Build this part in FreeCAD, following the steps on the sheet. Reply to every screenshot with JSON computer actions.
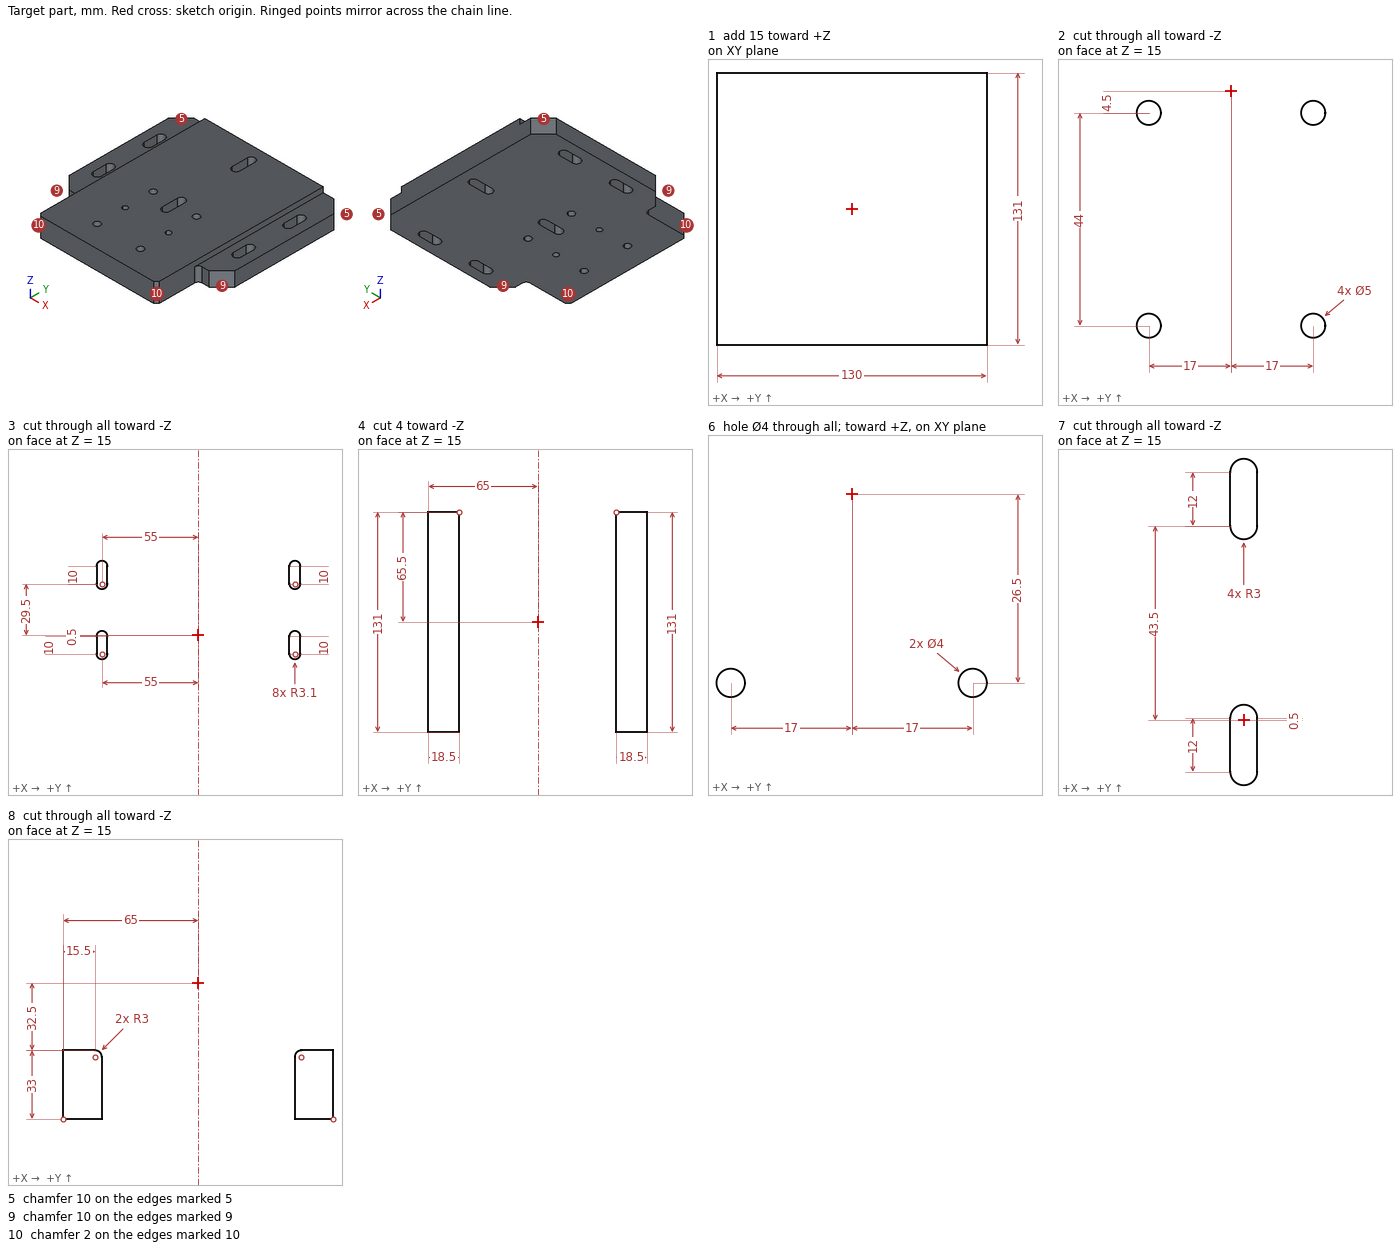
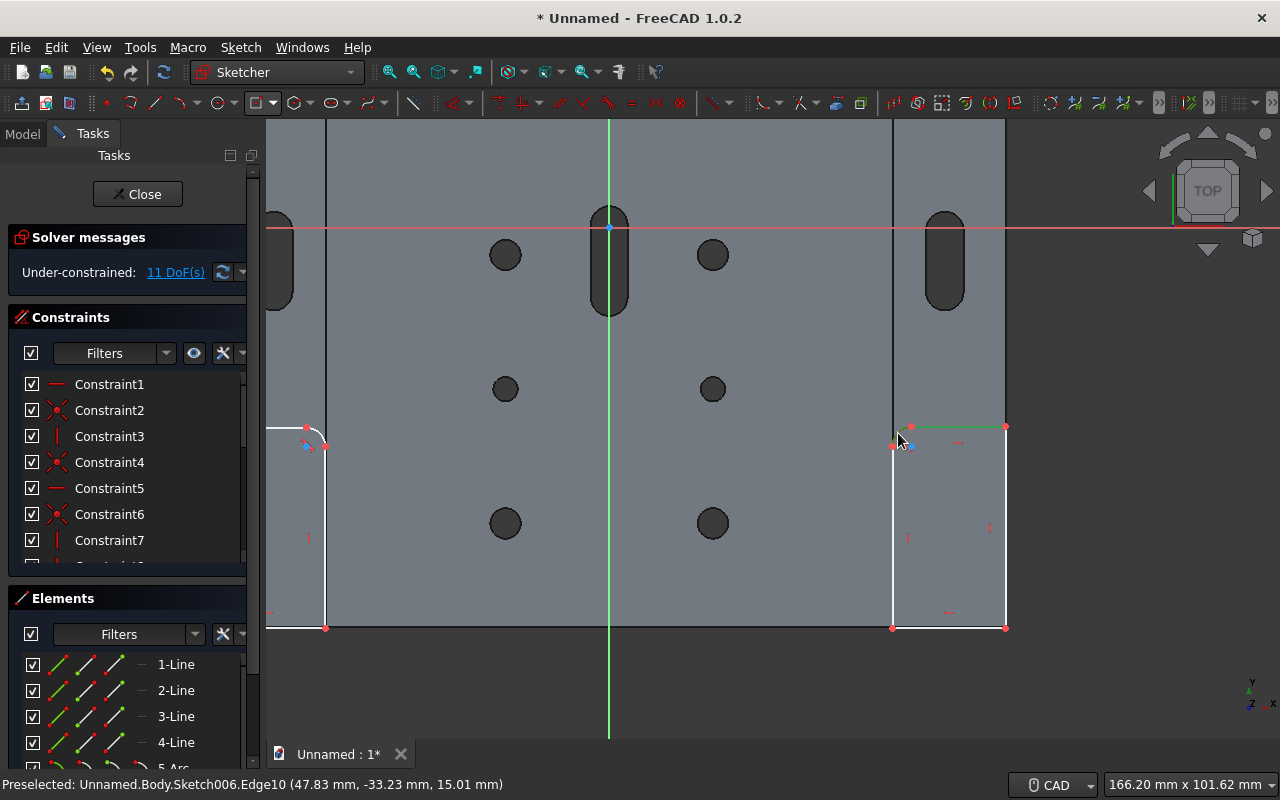
{"action": "key", "text": "t"}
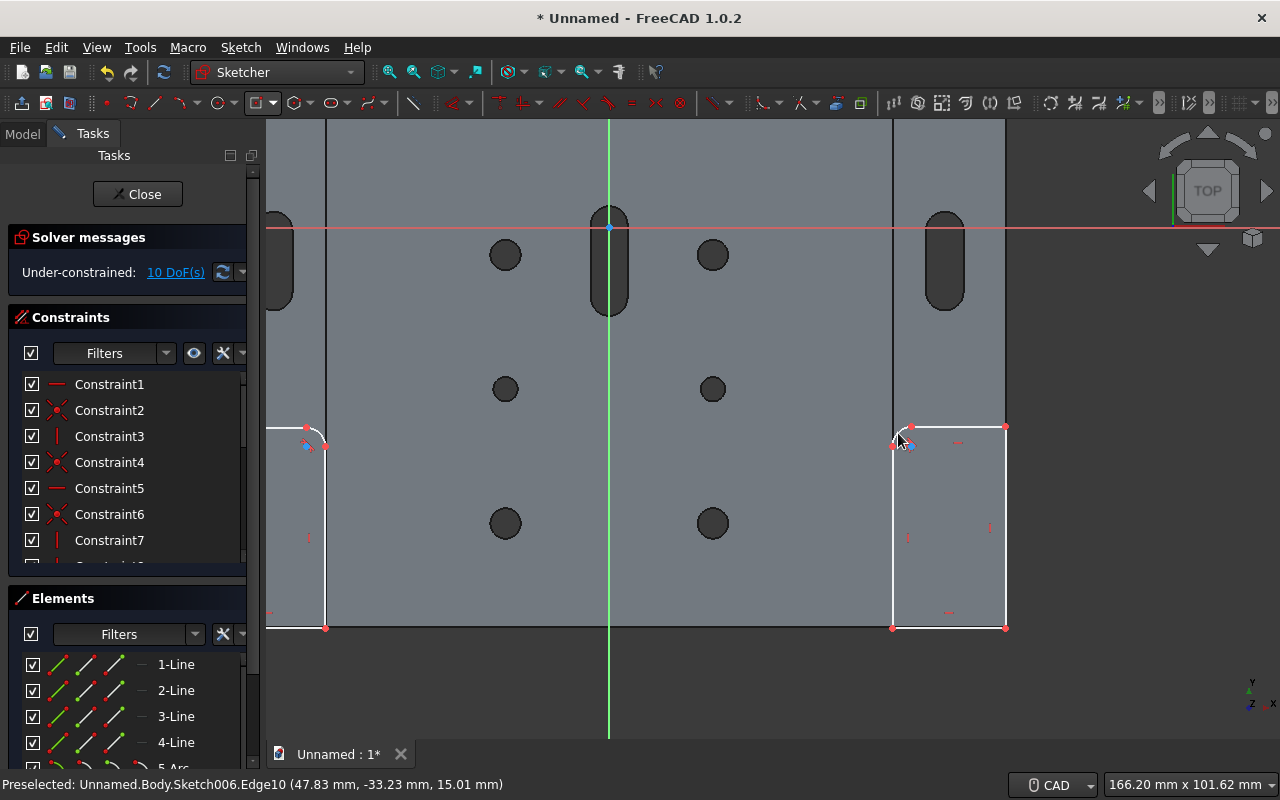
{"action": "left_click", "coordinate": [320, 433]}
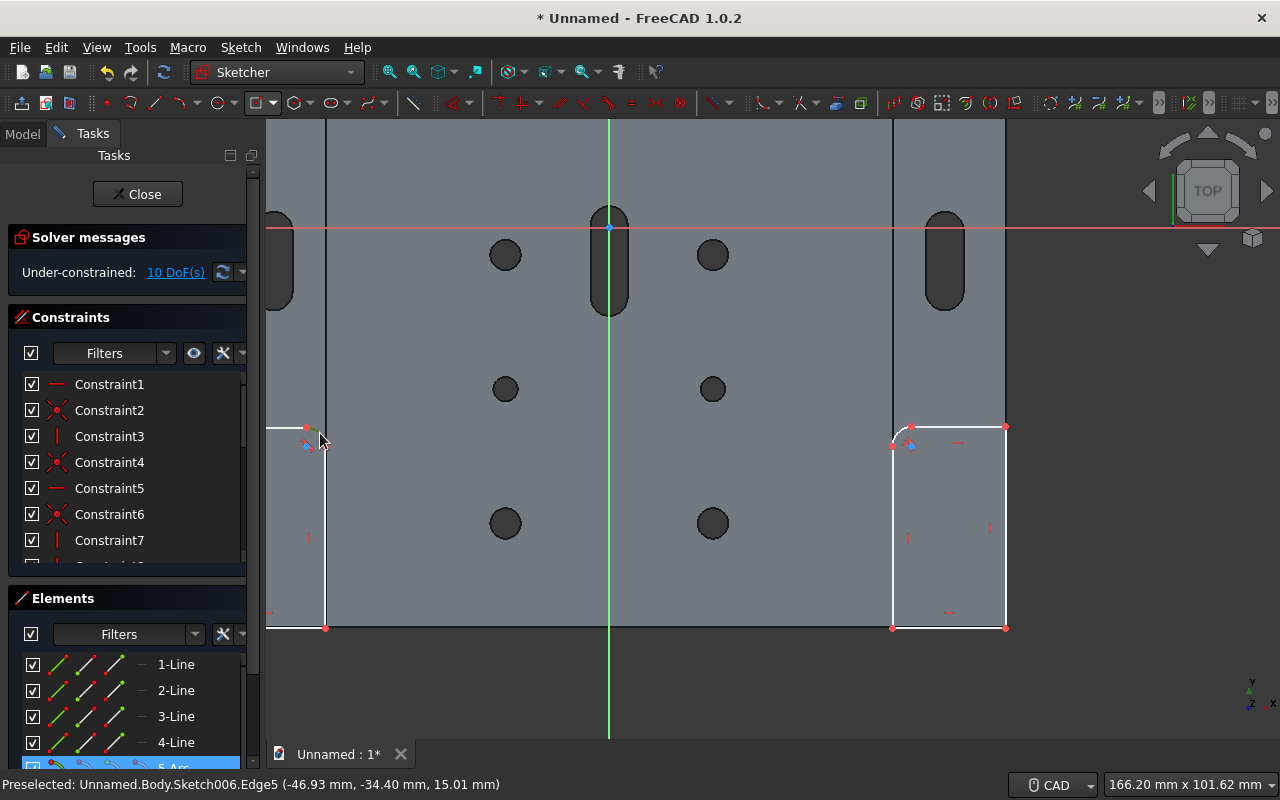
{"action": "scroll", "coordinate": [903, 429], "scroll_direction": "up", "scroll_amount": 3}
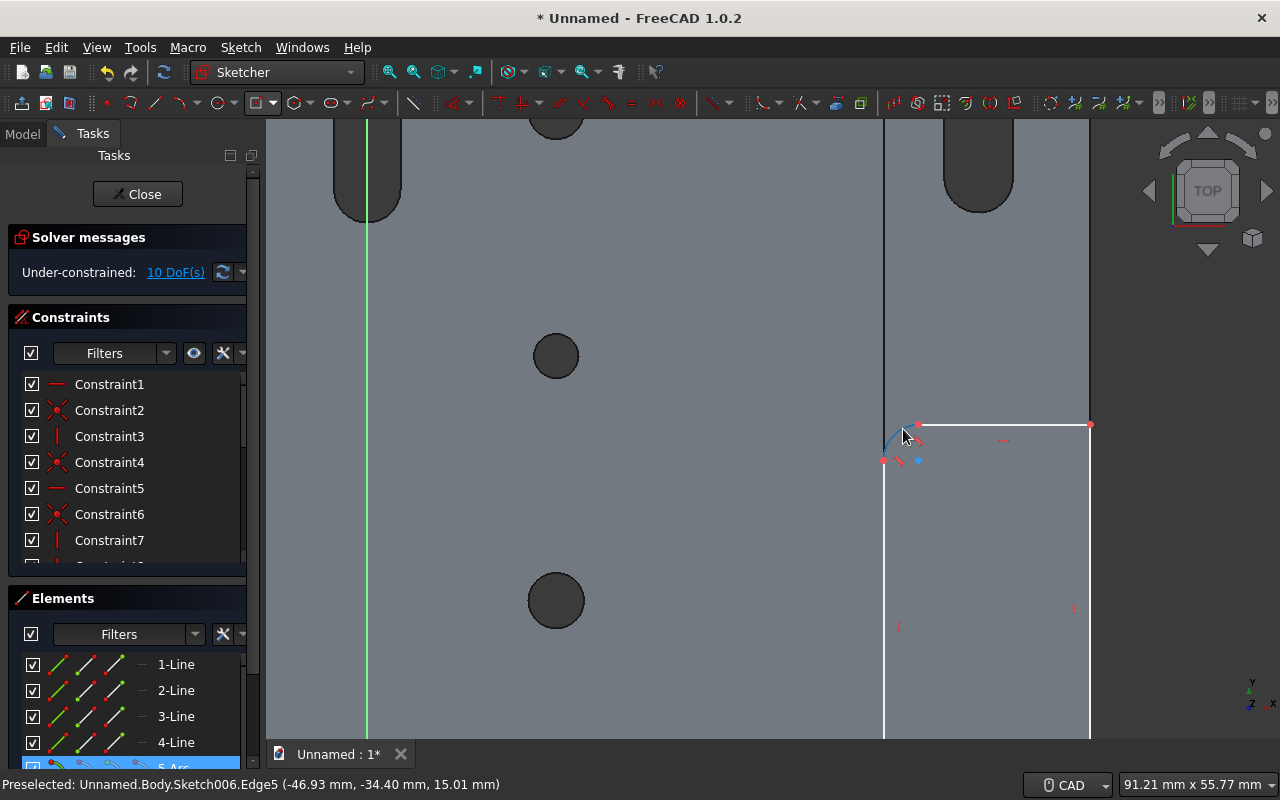
{"action": "left_click", "coordinate": [903, 429]}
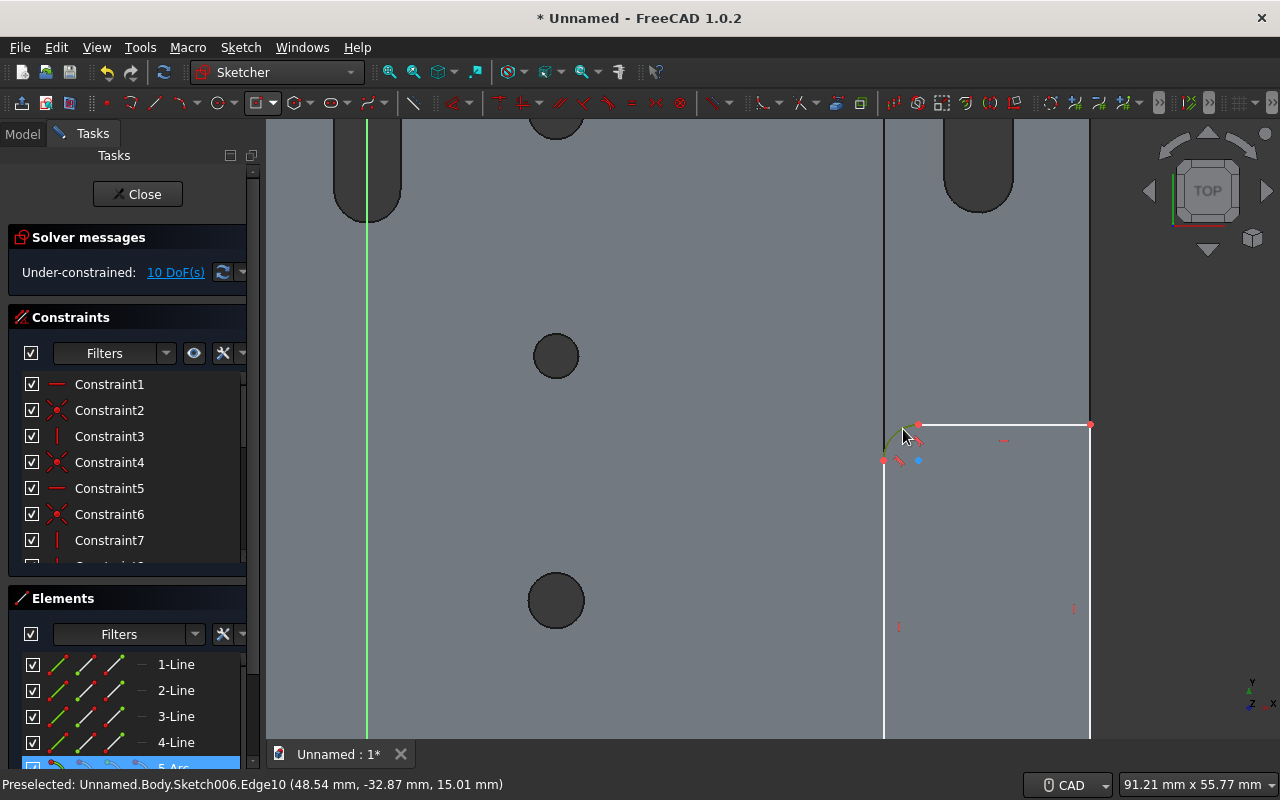
{"action": "key", "text": "e"}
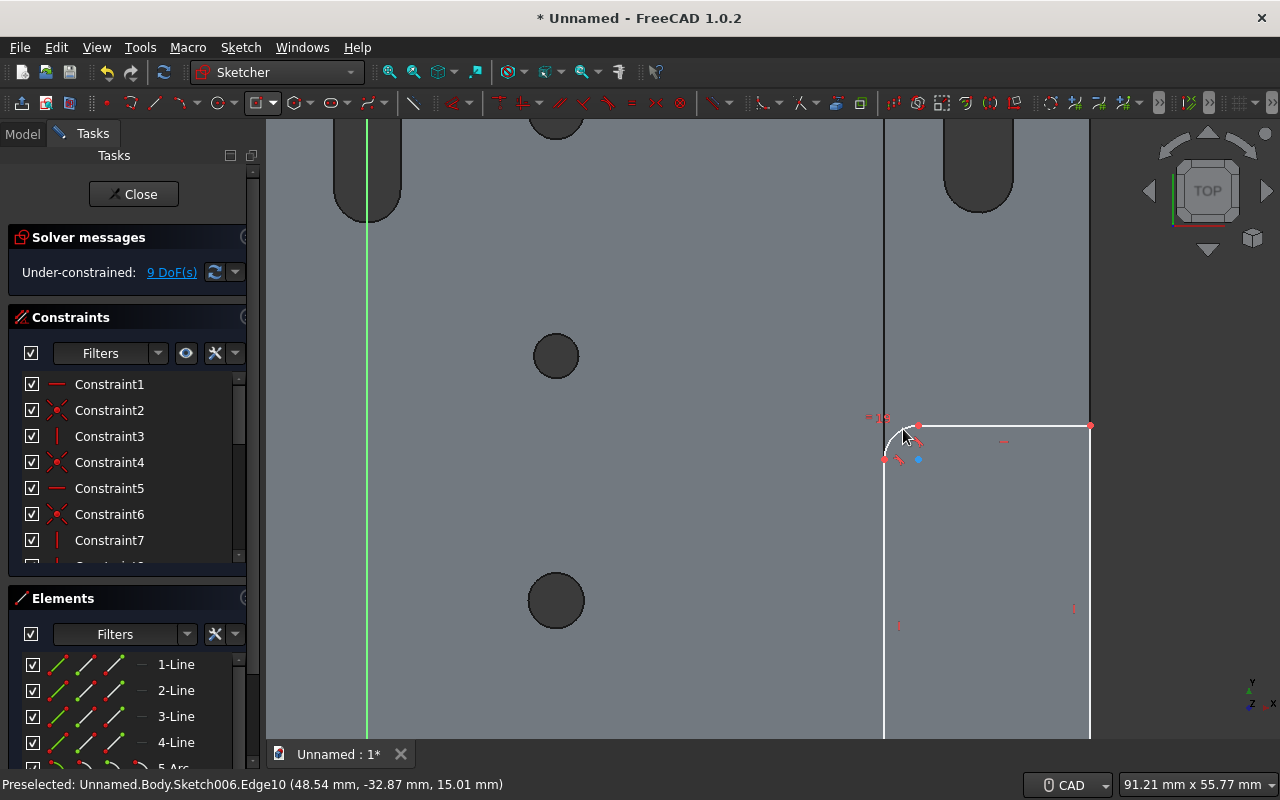
{"action": "scroll", "coordinate": [901, 431], "scroll_direction": "down", "scroll_amount": 5}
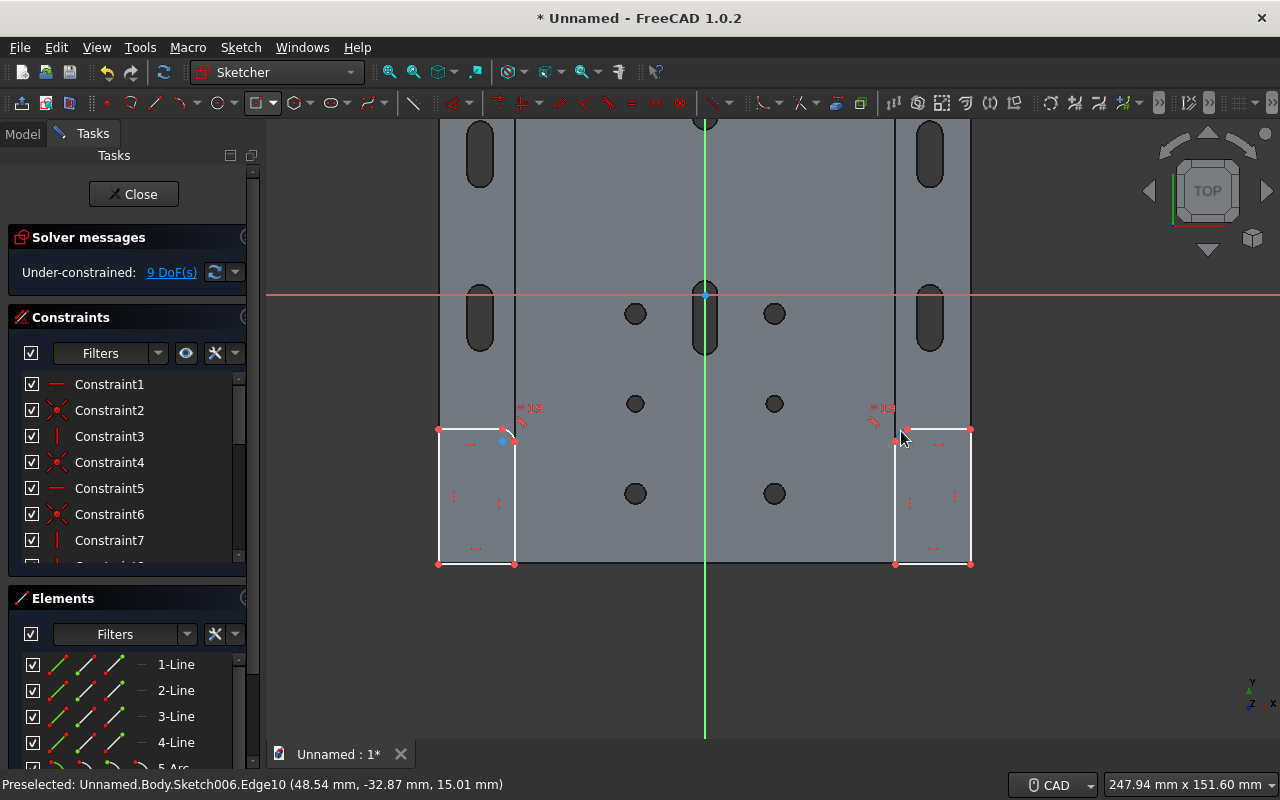
{"action": "left_click", "coordinate": [502, 442]}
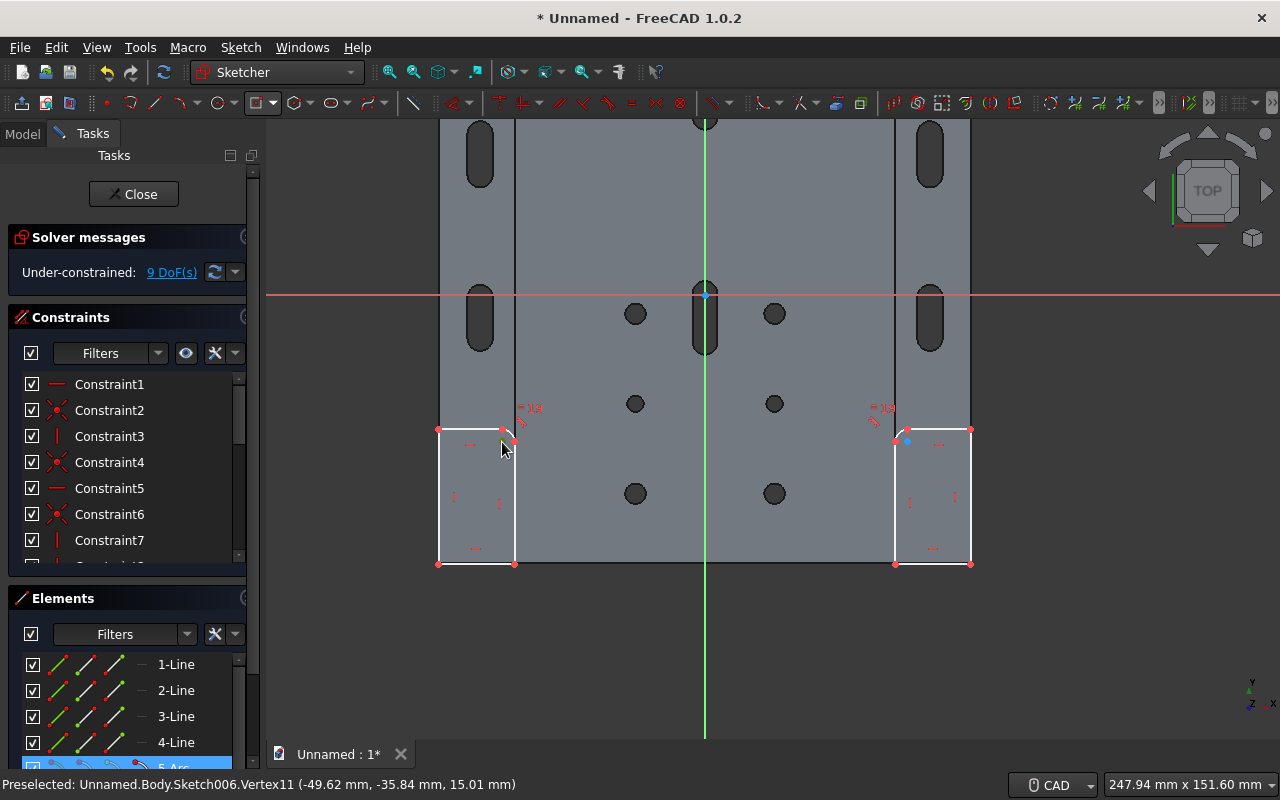
{"action": "left_click", "coordinate": [908, 442]}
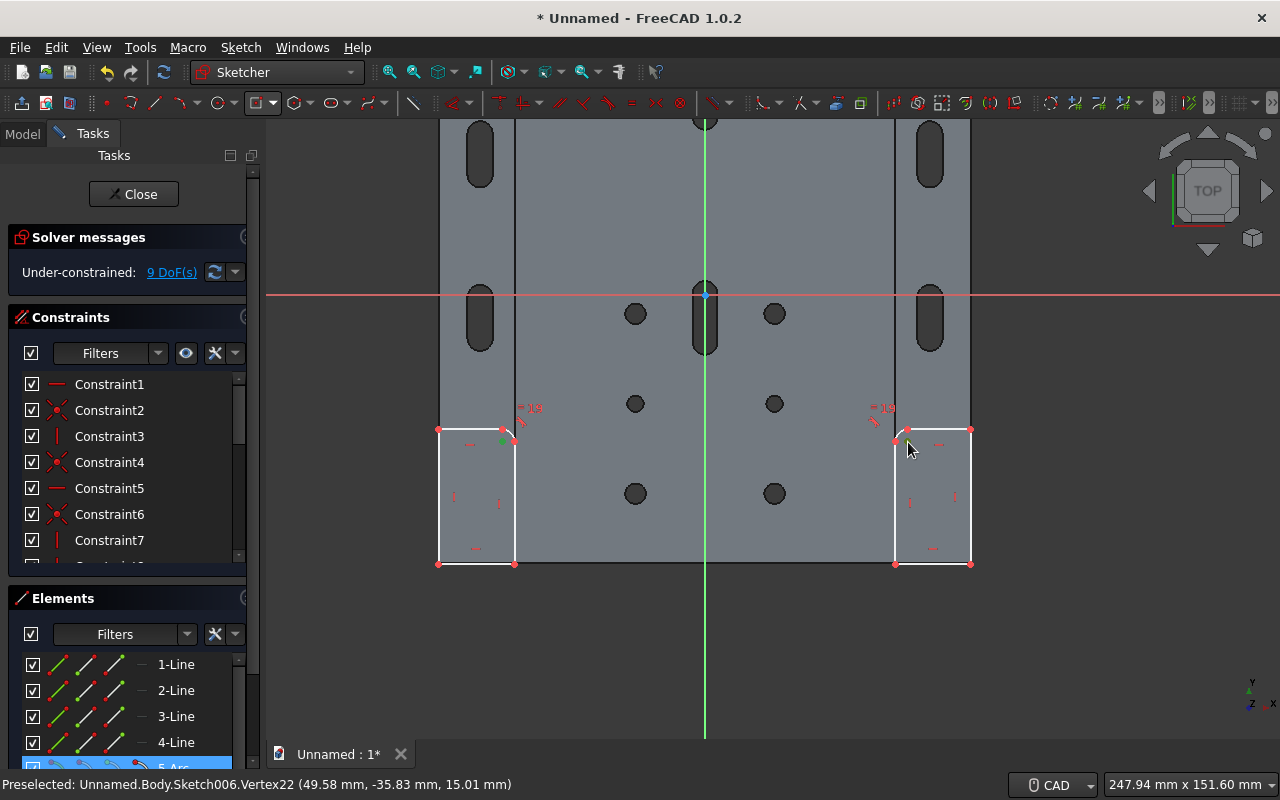
{"action": "left_click", "coordinate": [705, 671]}